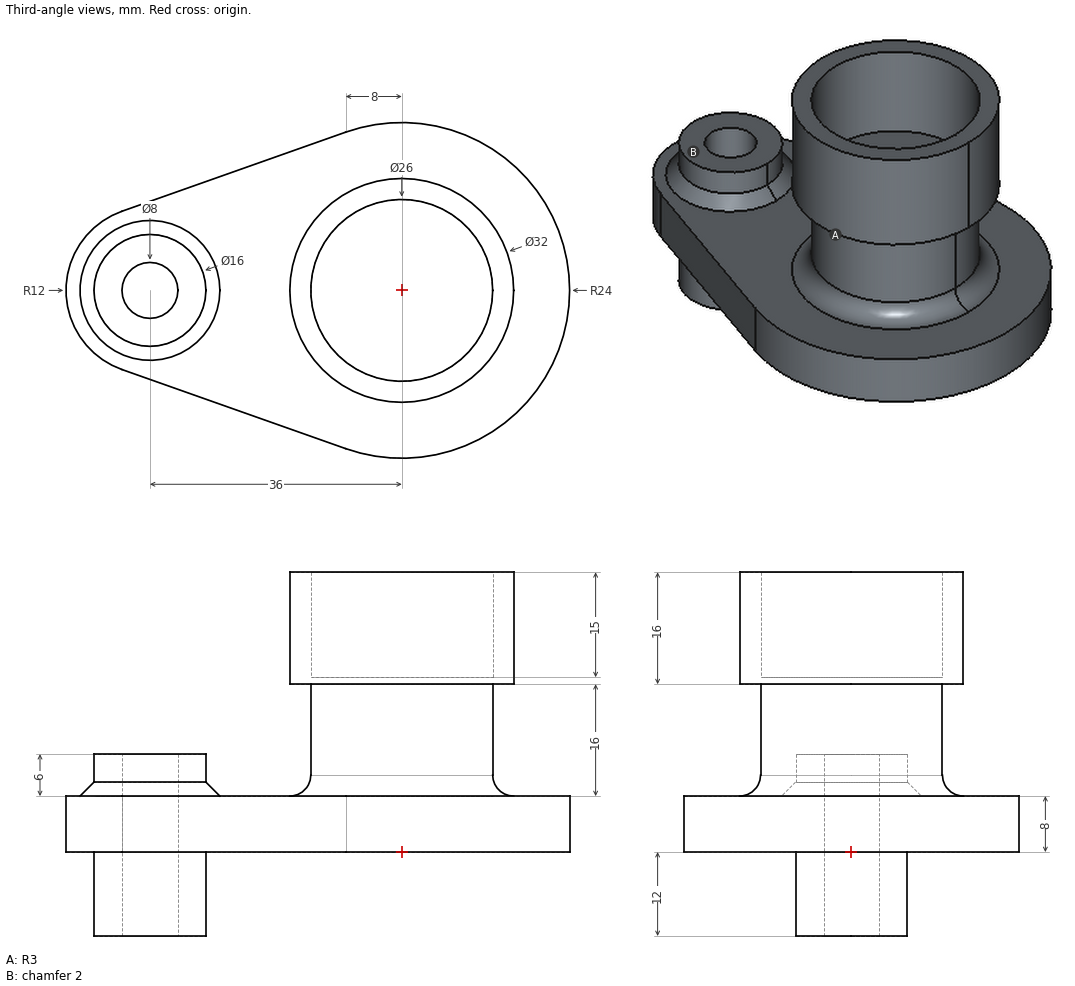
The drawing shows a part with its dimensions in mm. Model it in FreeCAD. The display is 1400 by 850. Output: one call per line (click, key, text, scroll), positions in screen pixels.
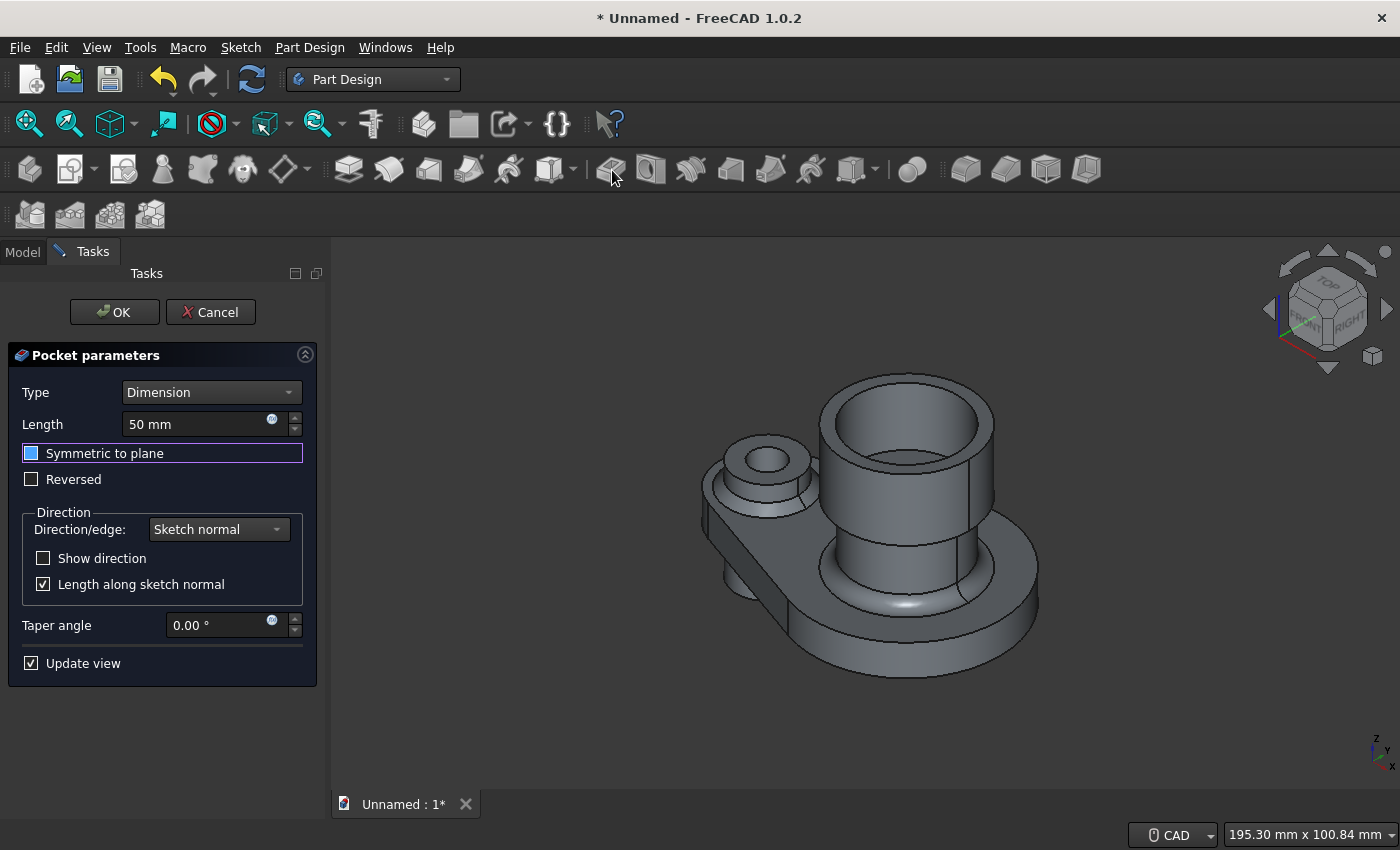
click(115, 312)